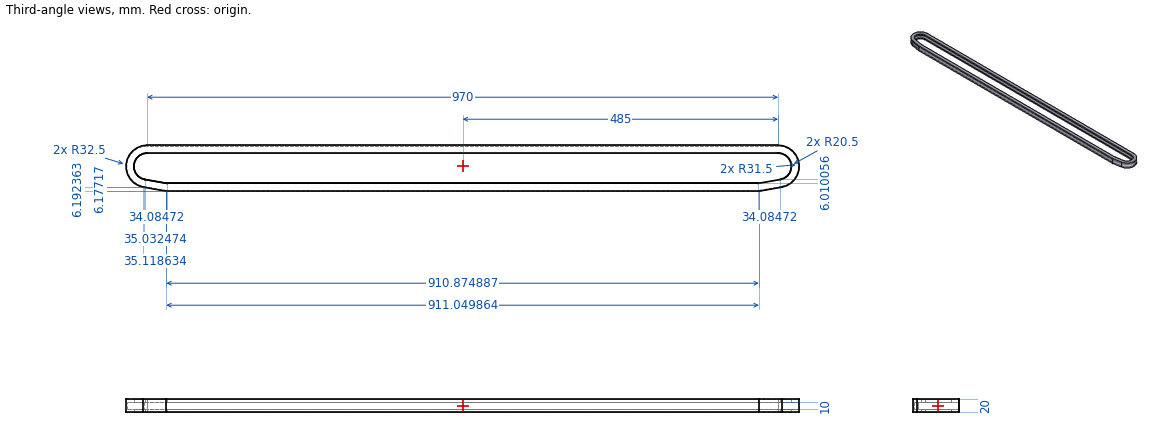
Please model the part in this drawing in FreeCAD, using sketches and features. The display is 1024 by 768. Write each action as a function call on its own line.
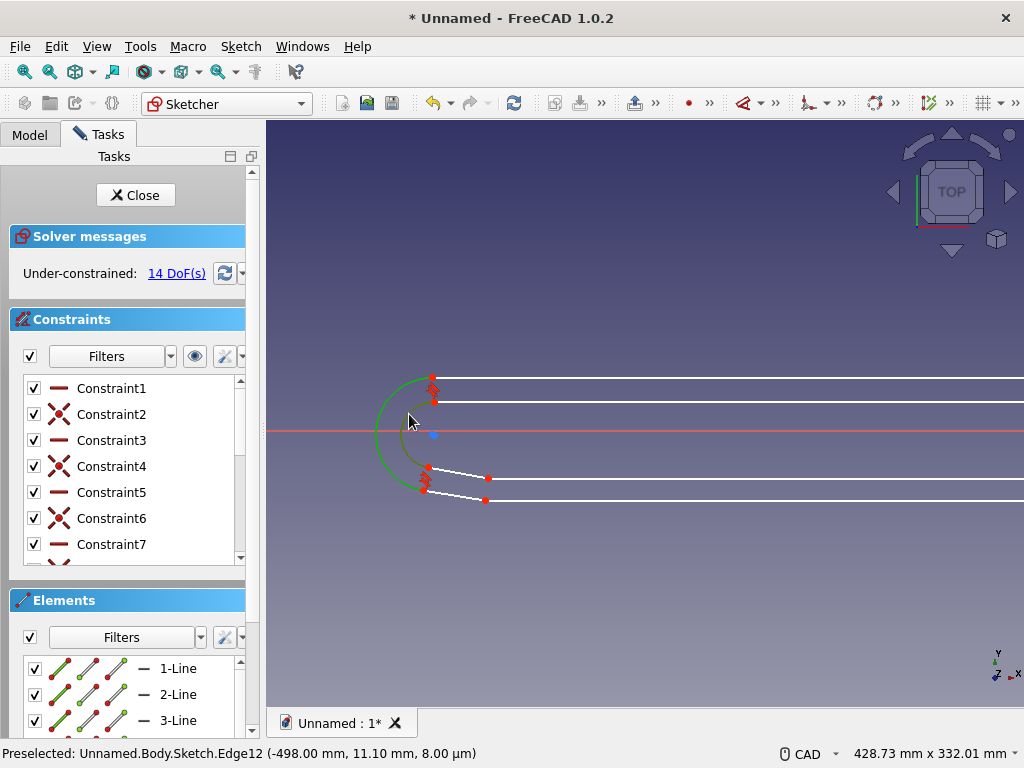
key(c)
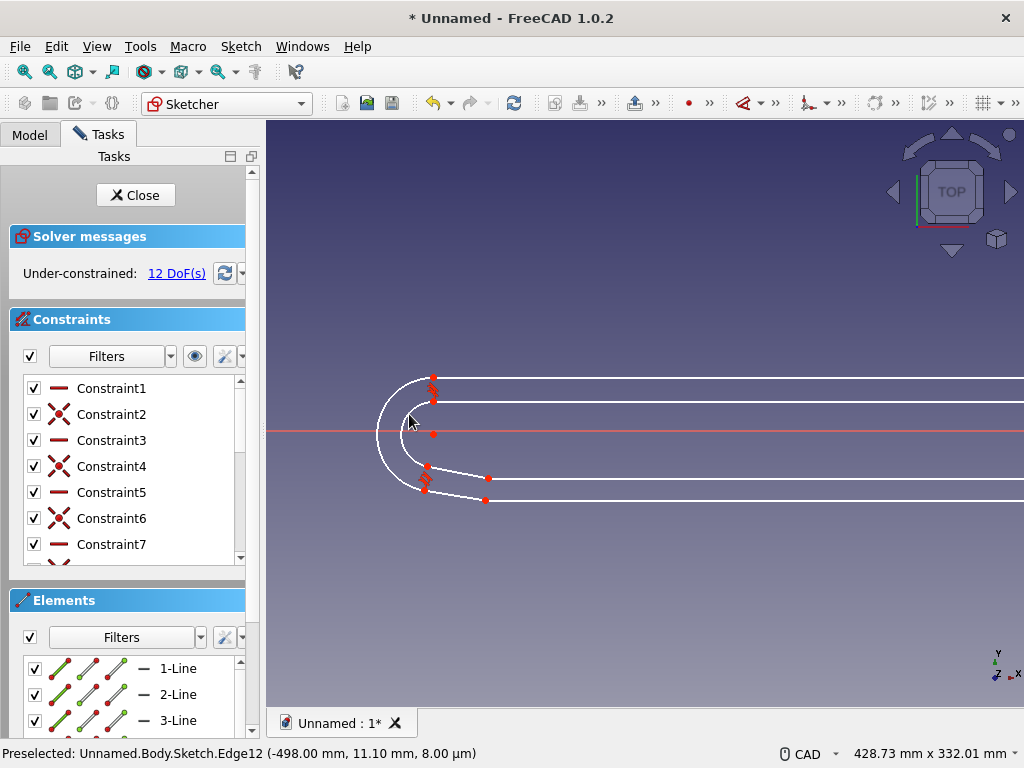
click(390, 399)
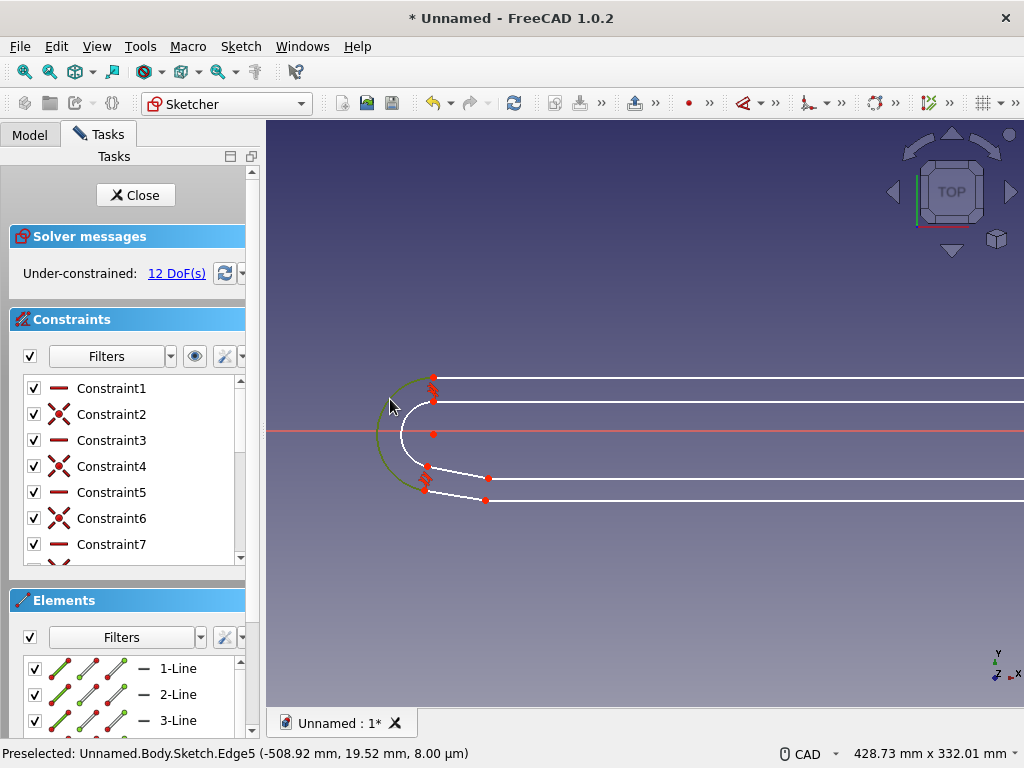
scroll(396, 408, down, 8)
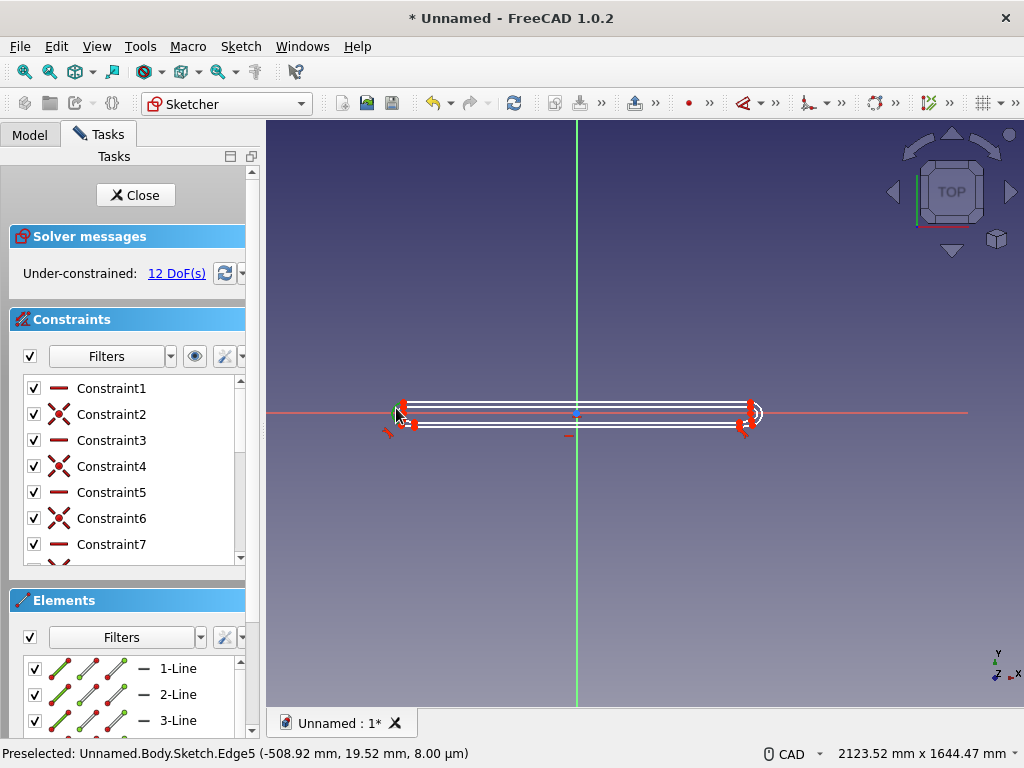
scroll(760, 420, up, 6)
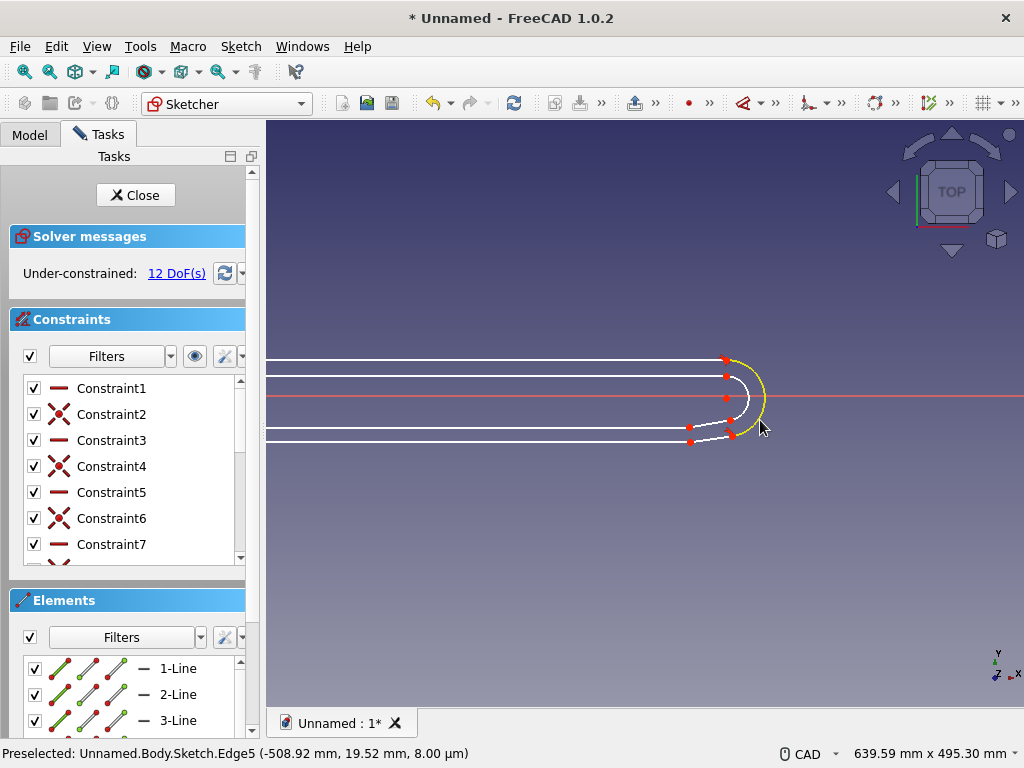
click(760, 418)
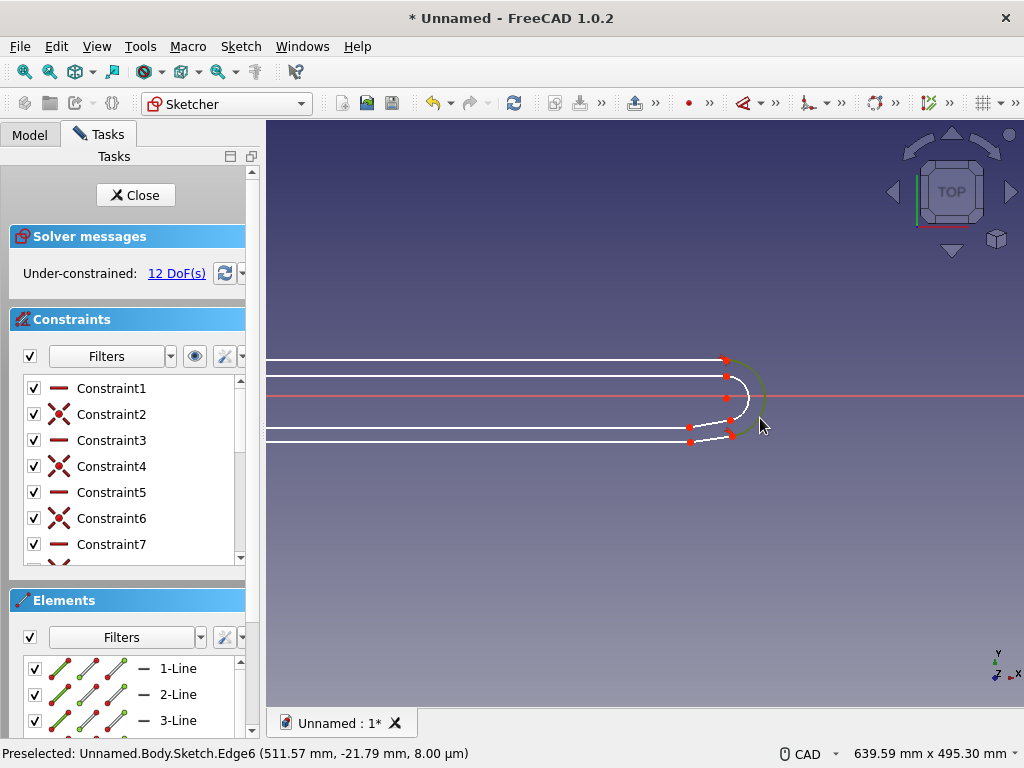
key(e)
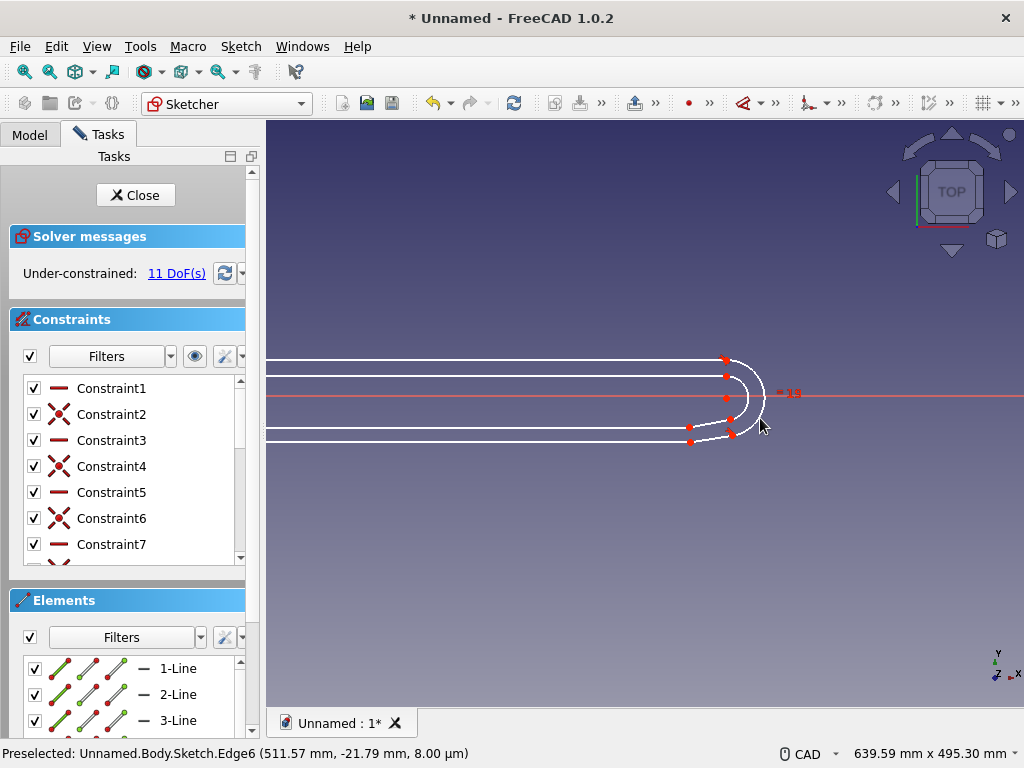
scroll(760, 420, down, 6)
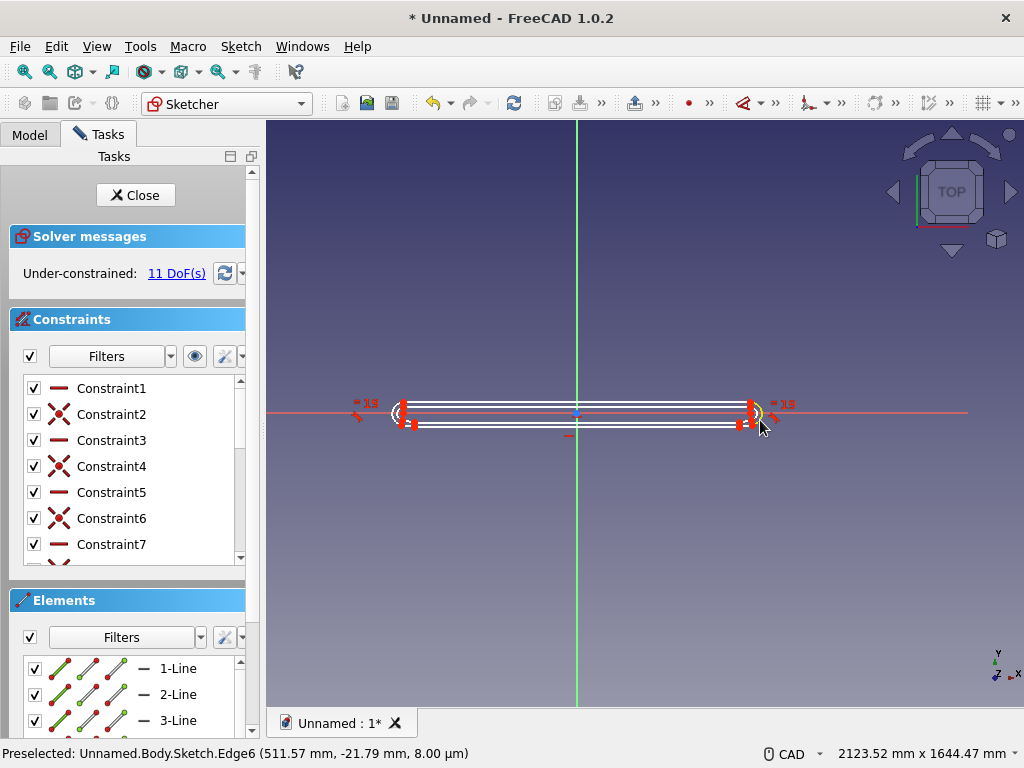
scroll(404, 414, up, 4)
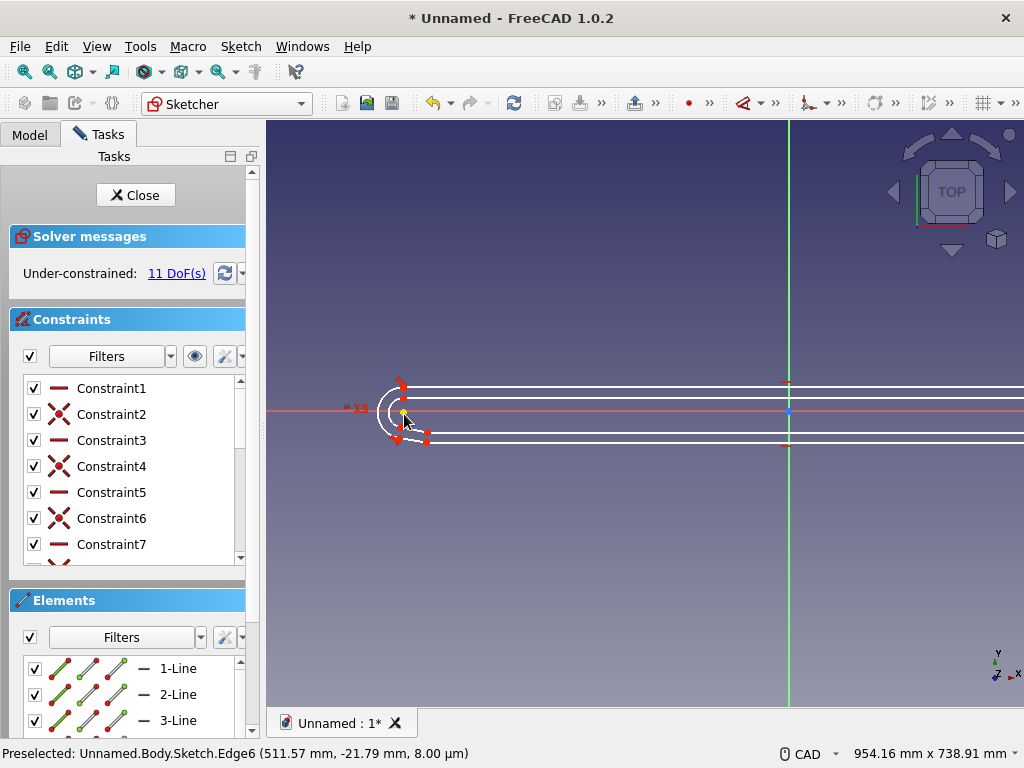
click(403, 413)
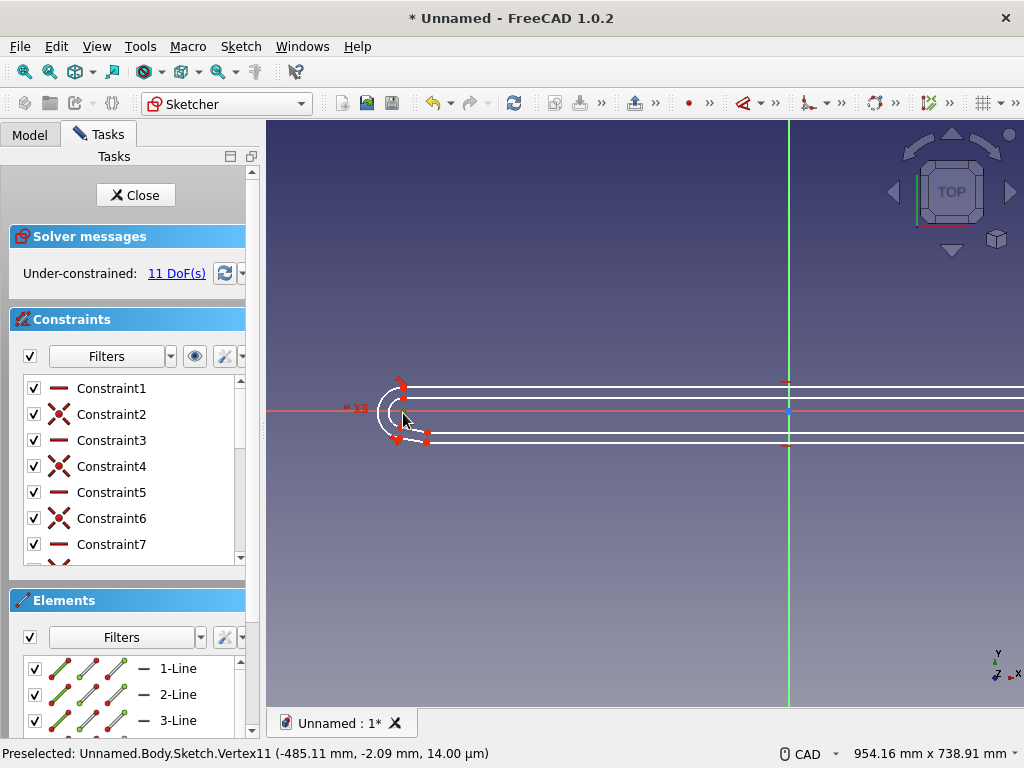
click(334, 411)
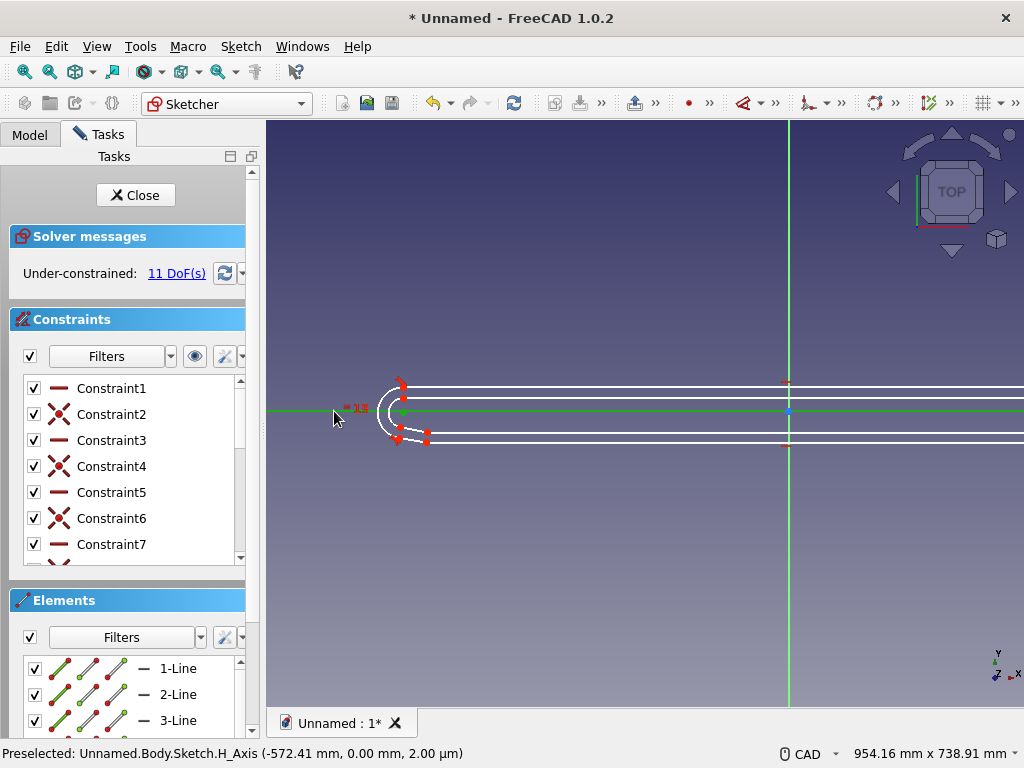
key(c)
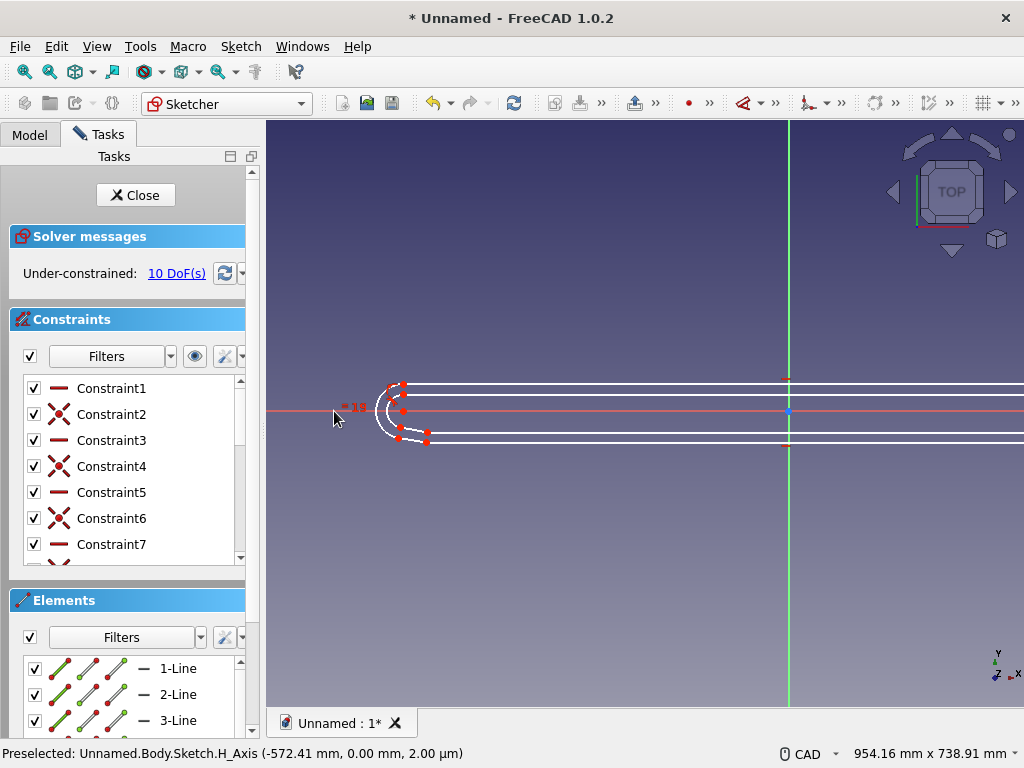
key(d)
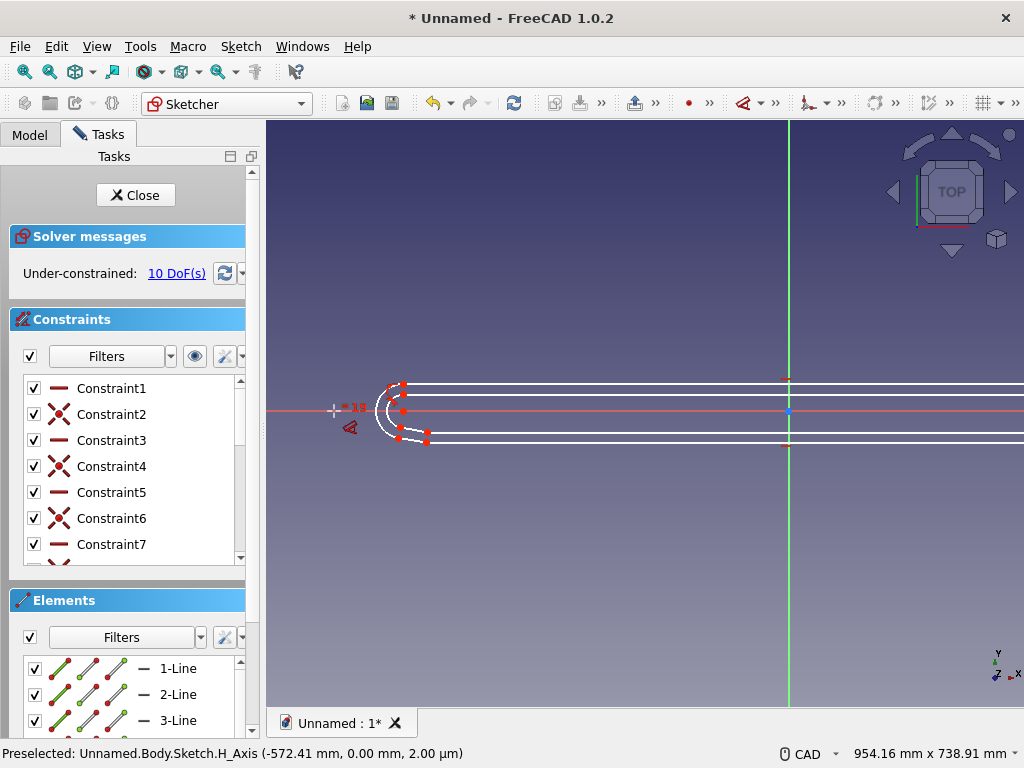
scroll(382, 394, up, 3)